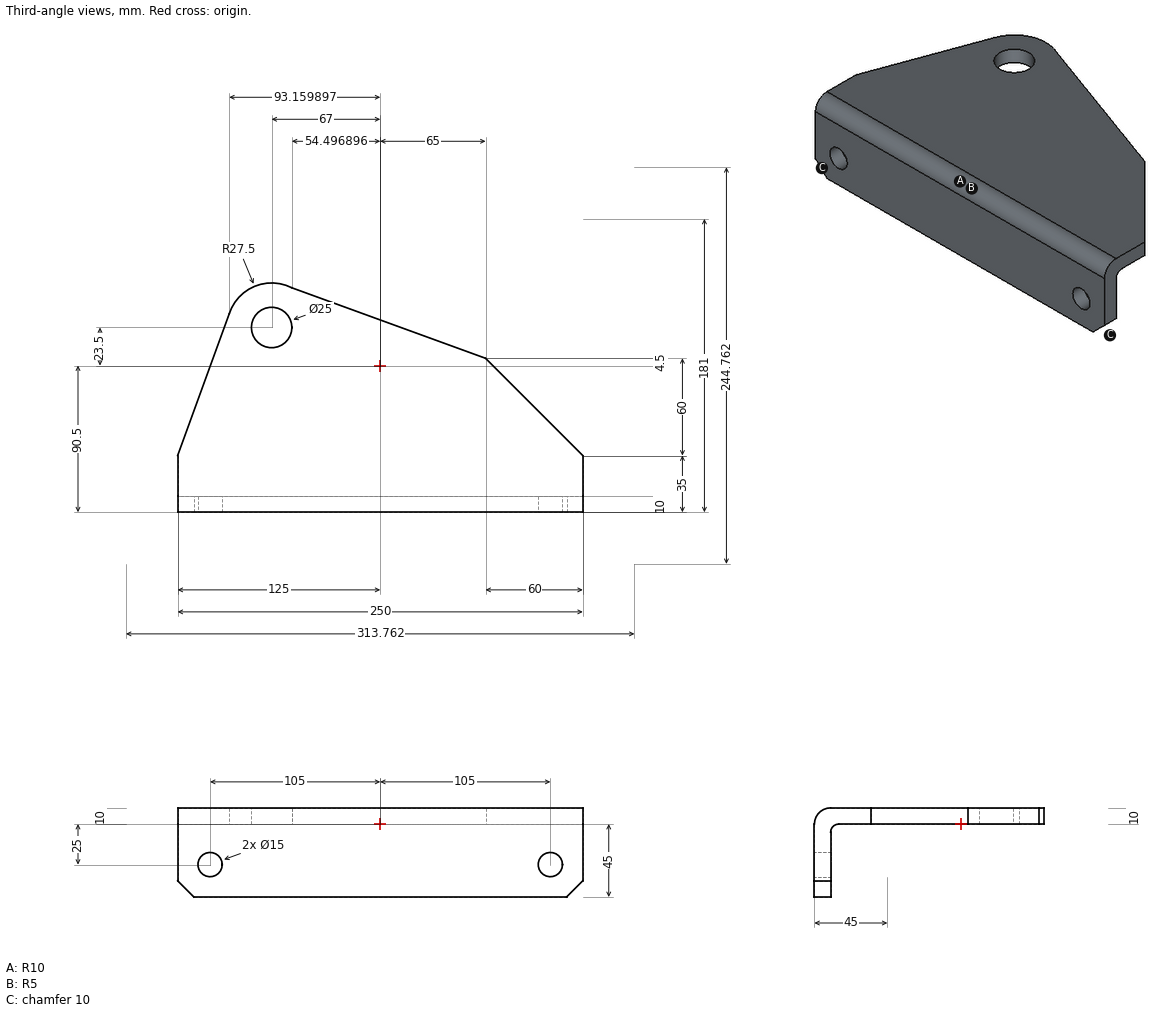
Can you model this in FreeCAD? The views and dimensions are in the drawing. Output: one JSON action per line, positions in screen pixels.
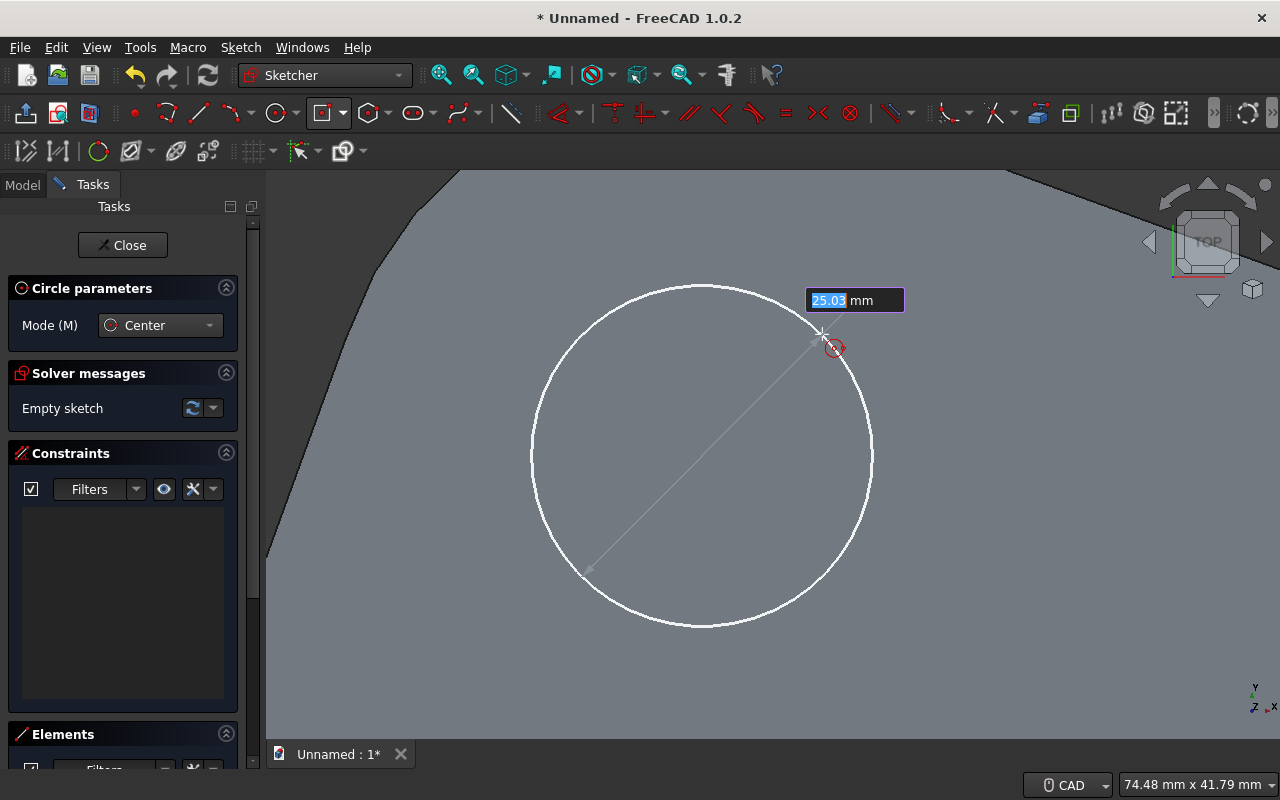
{"action": "type", "text": "25"}
{"action": "key", "text": "Return"}
{"action": "key", "text": "Escape"}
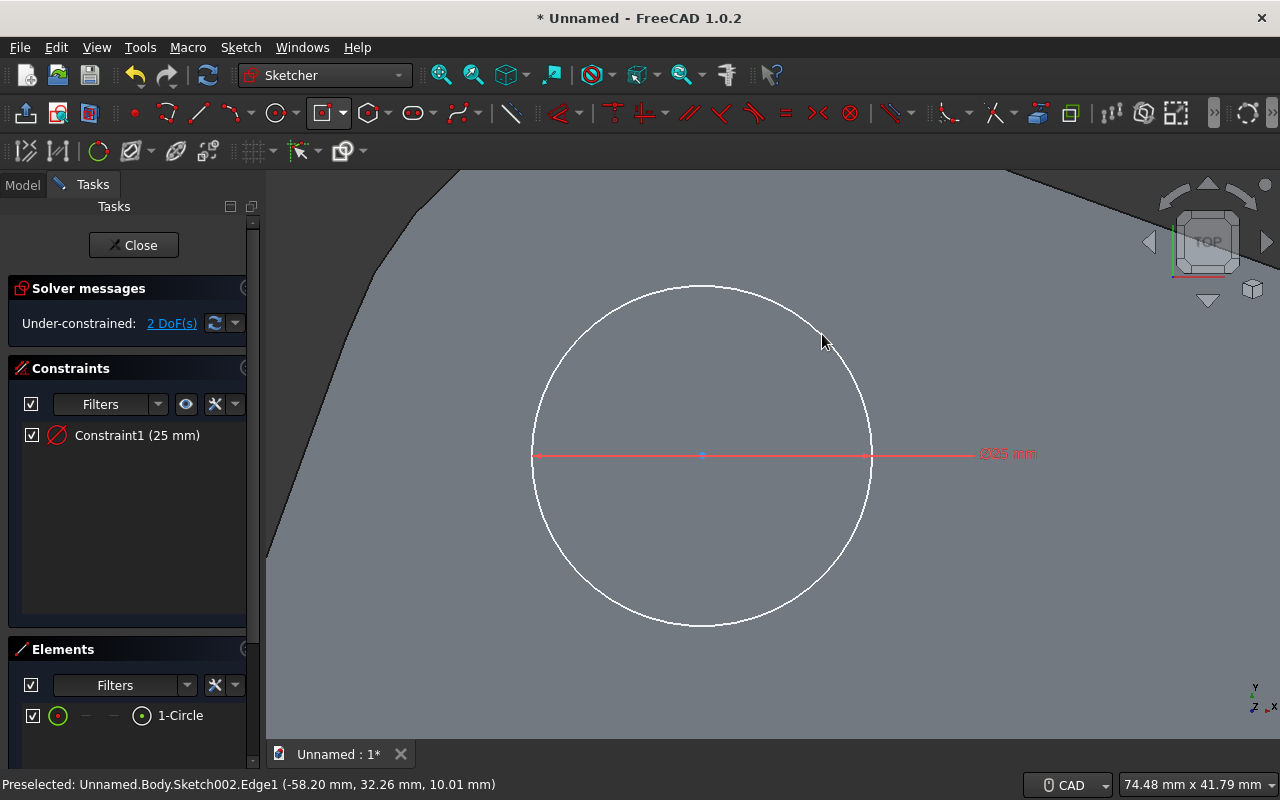
{"action": "left_click", "coordinate": [558, 114]}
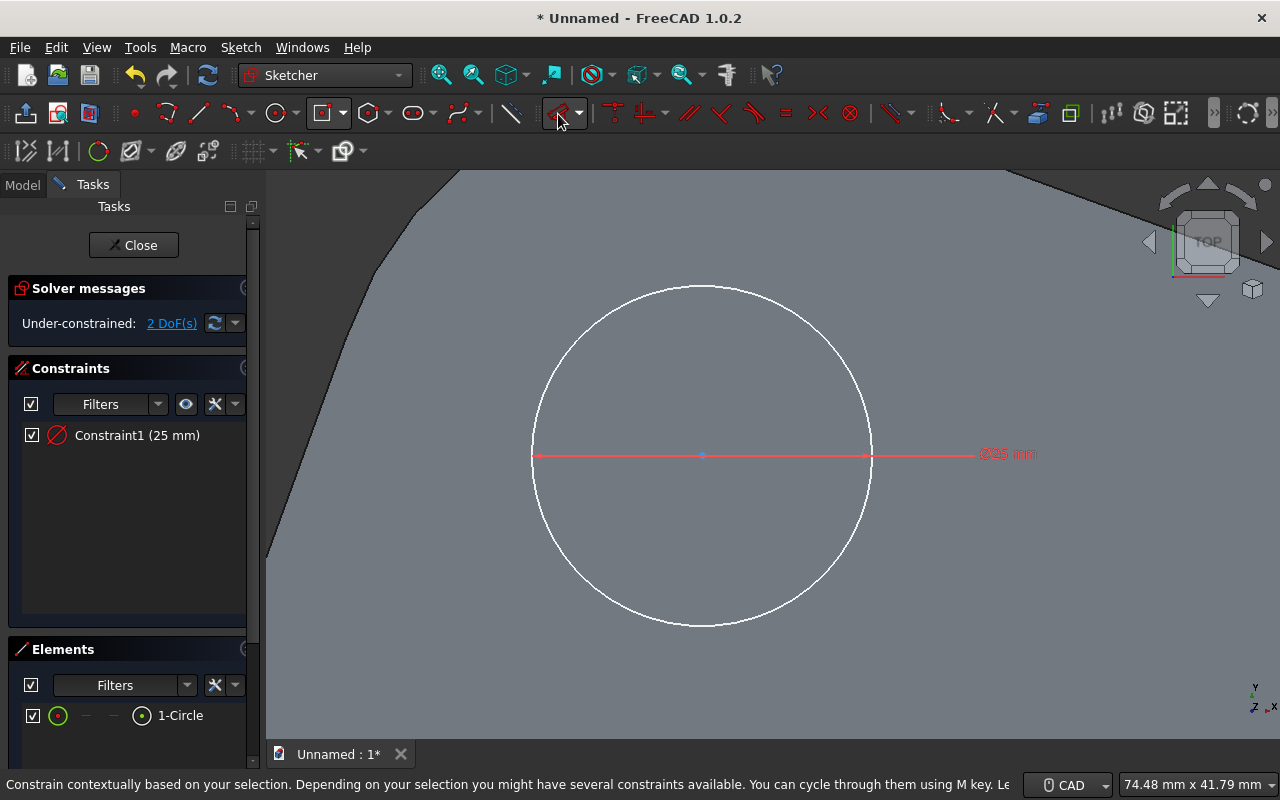
{"action": "left_click", "coordinate": [702, 456]}
{"action": "left_click", "coordinate": [909, 422]}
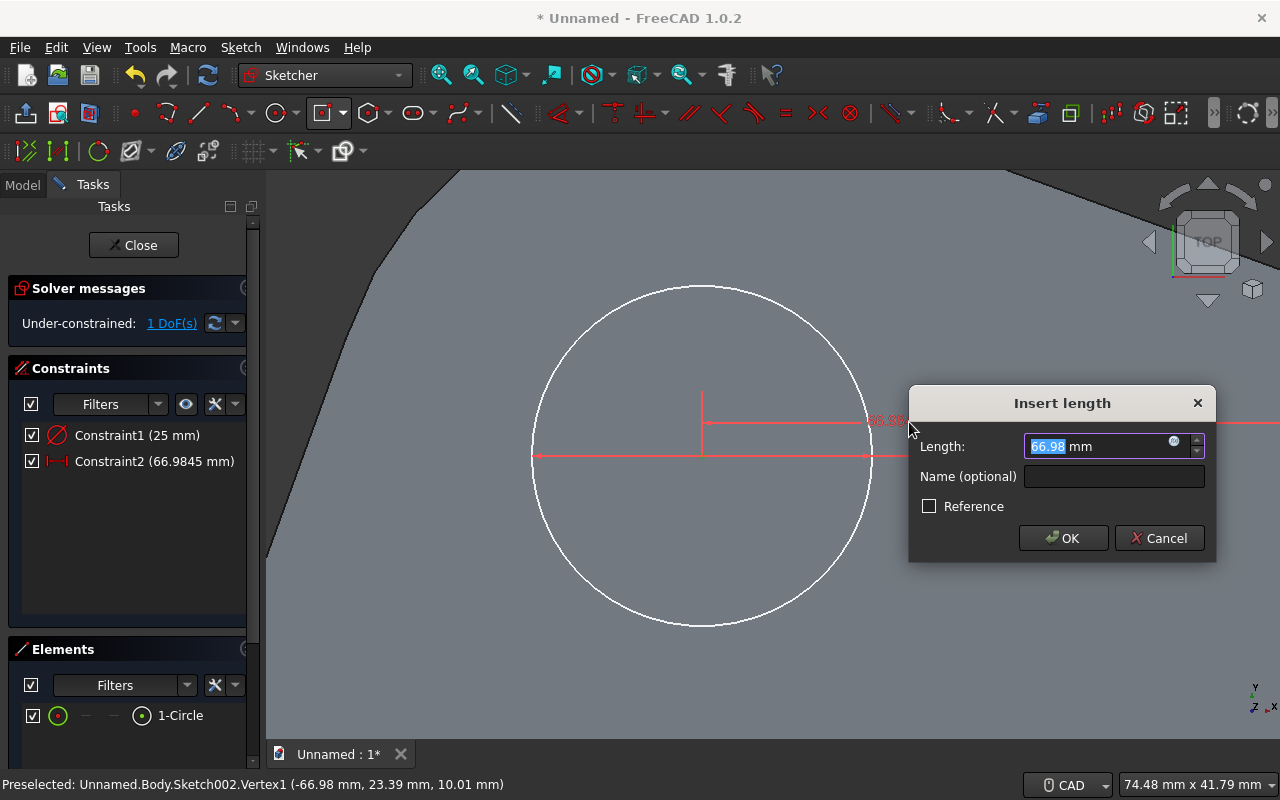
{"action": "type", "text": "67"}
{"action": "key", "text": "Return"}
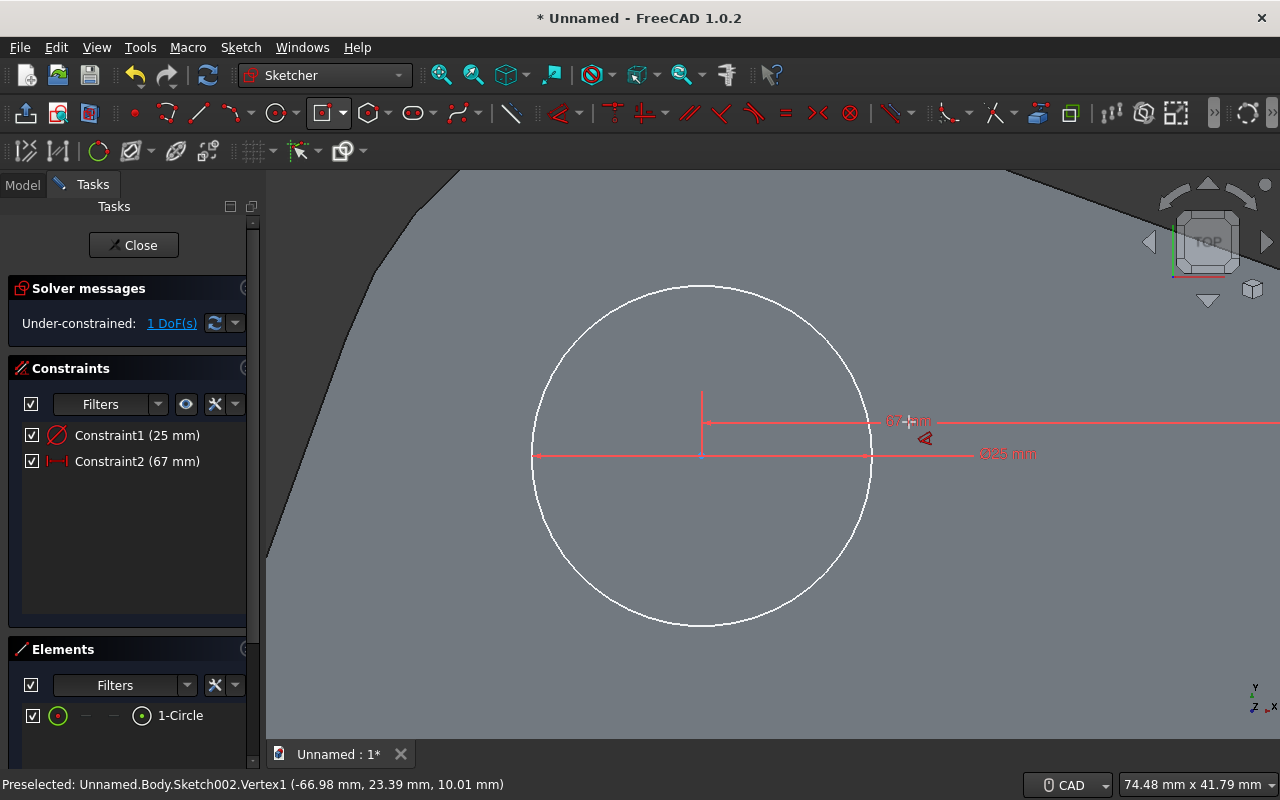
{"action": "left_click", "coordinate": [702, 456]}
{"action": "left_click", "coordinate": [668, 583]}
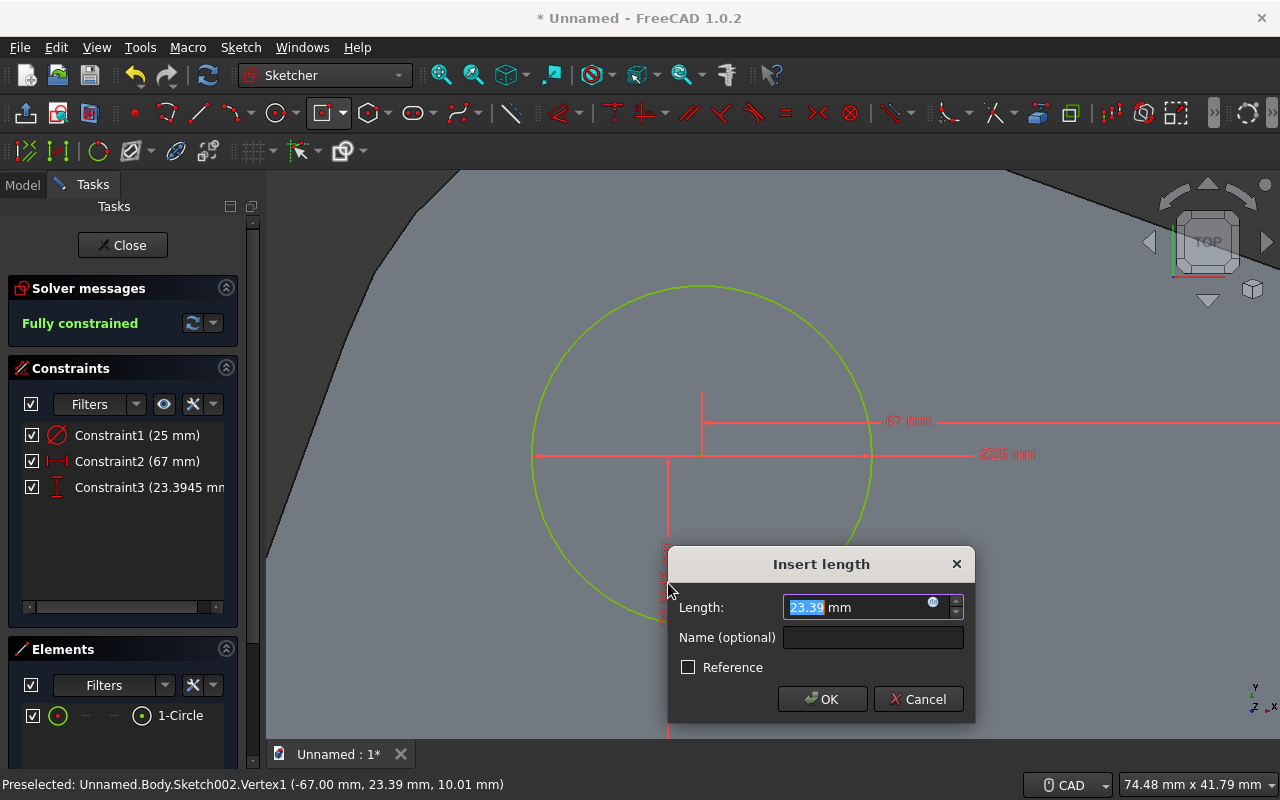
{"action": "type", "text": "23.5"}
{"action": "key", "text": "Return"}
{"action": "key", "text": "Escape"}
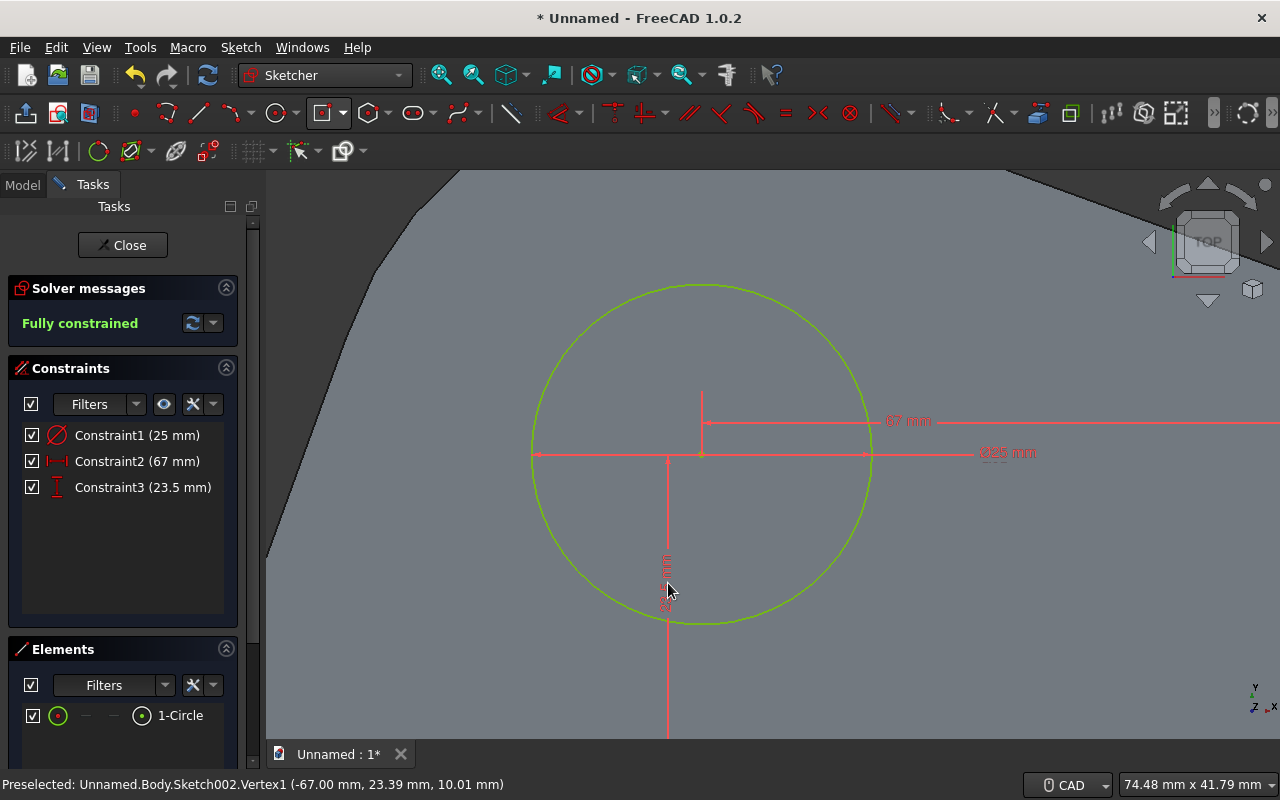
{"action": "left_click", "coordinate": [123, 245]}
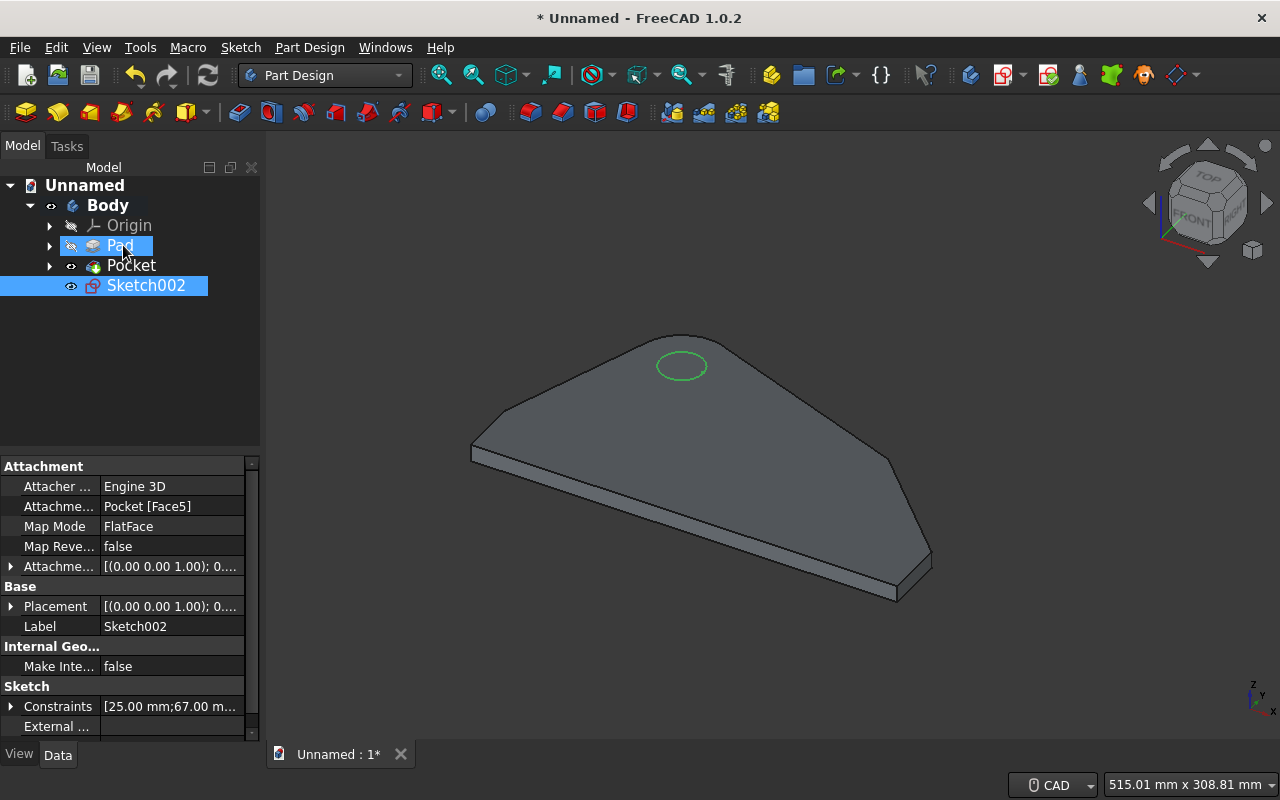
{"action": "left_click", "coordinate": [240, 112]}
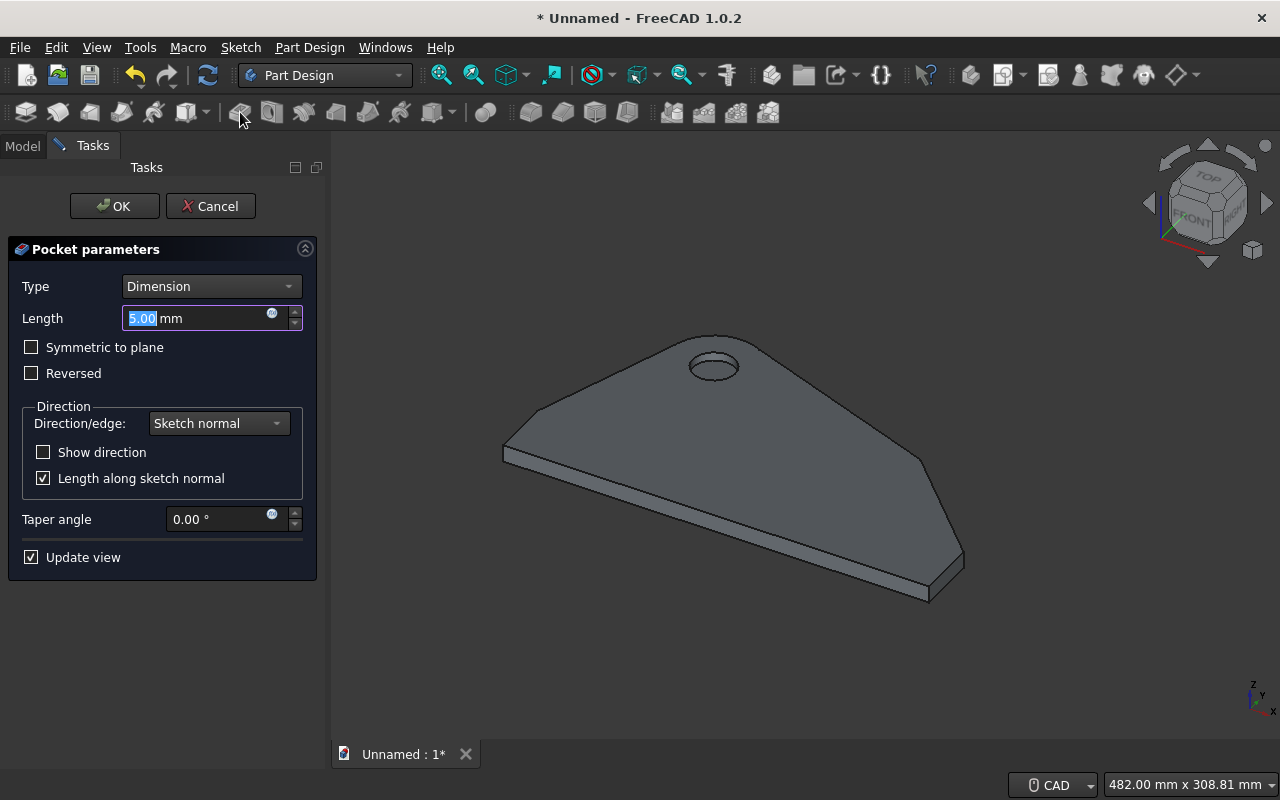
{"action": "type", "text": "10"}
{"action": "key", "text": "Tab"}